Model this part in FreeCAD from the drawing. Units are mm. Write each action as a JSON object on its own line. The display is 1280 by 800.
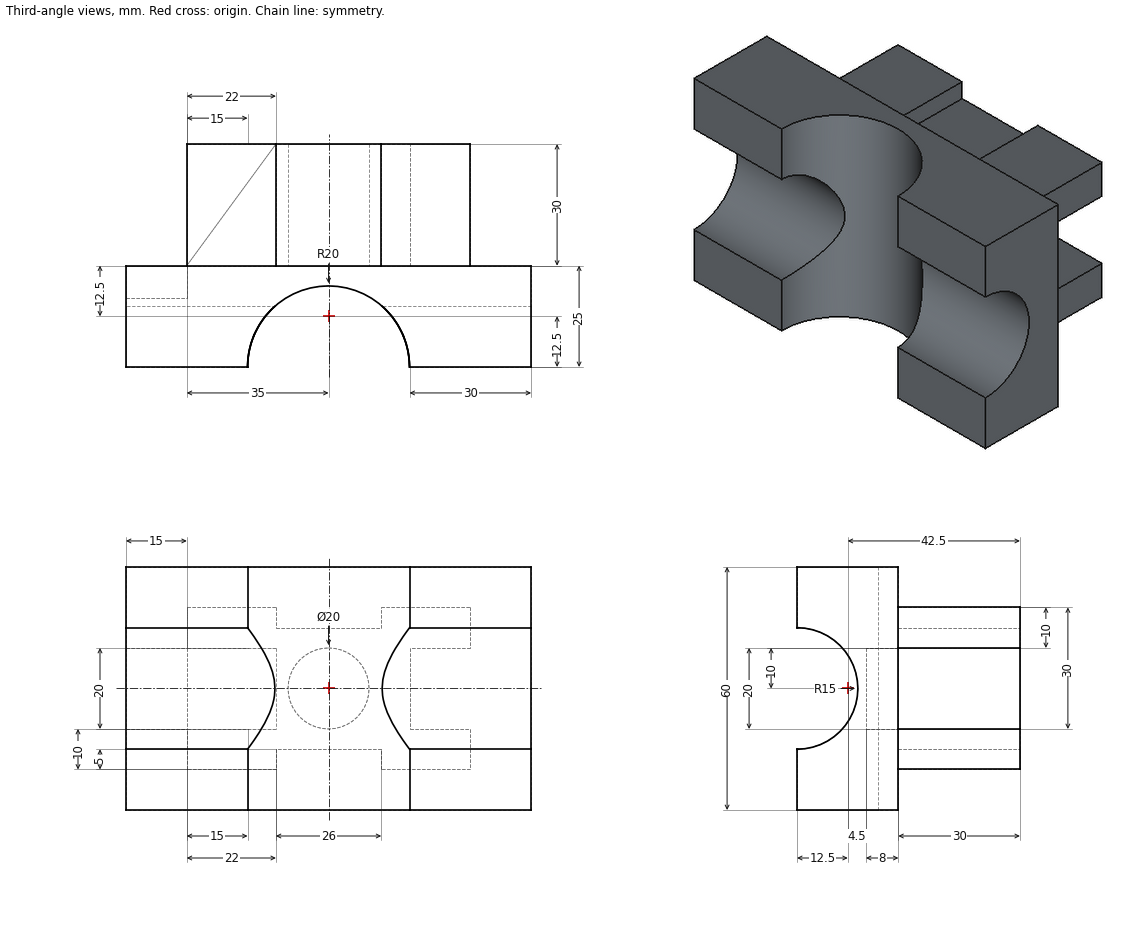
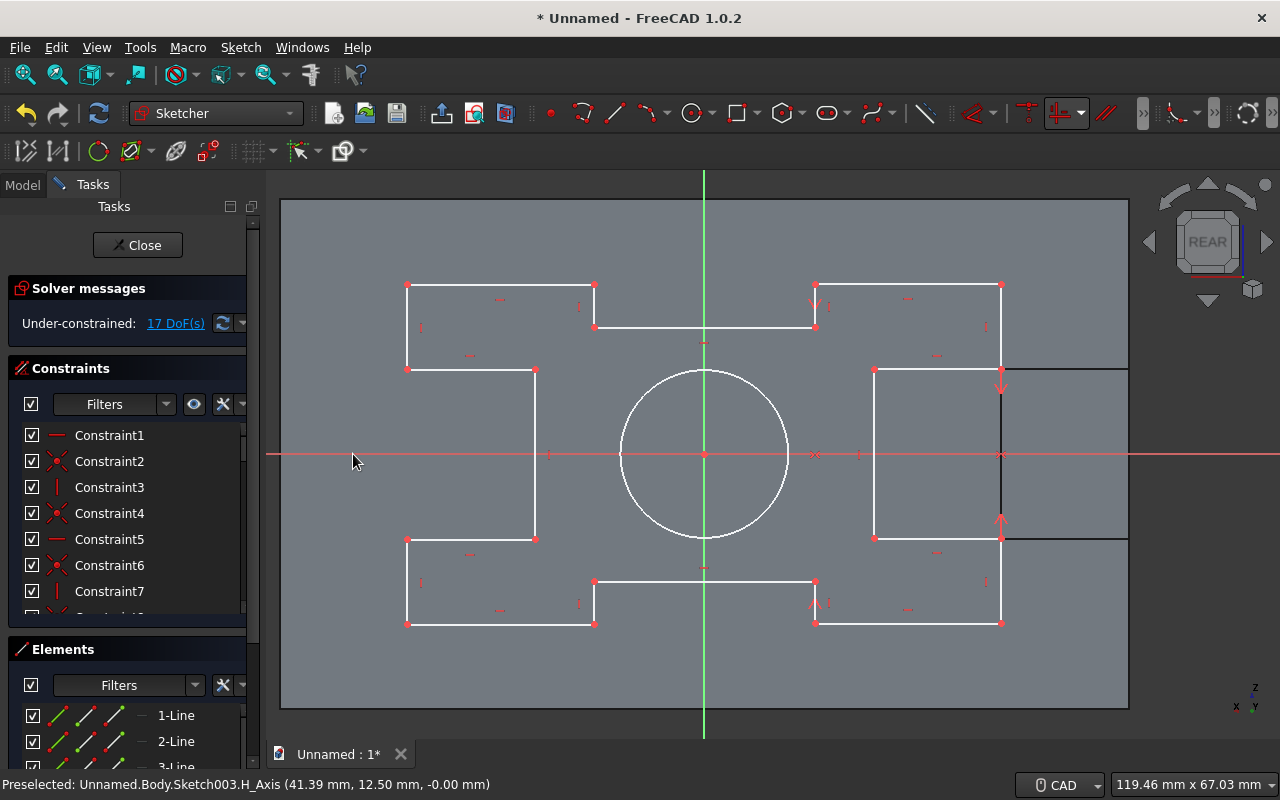
{"action": "left_click", "coordinate": [594, 582]}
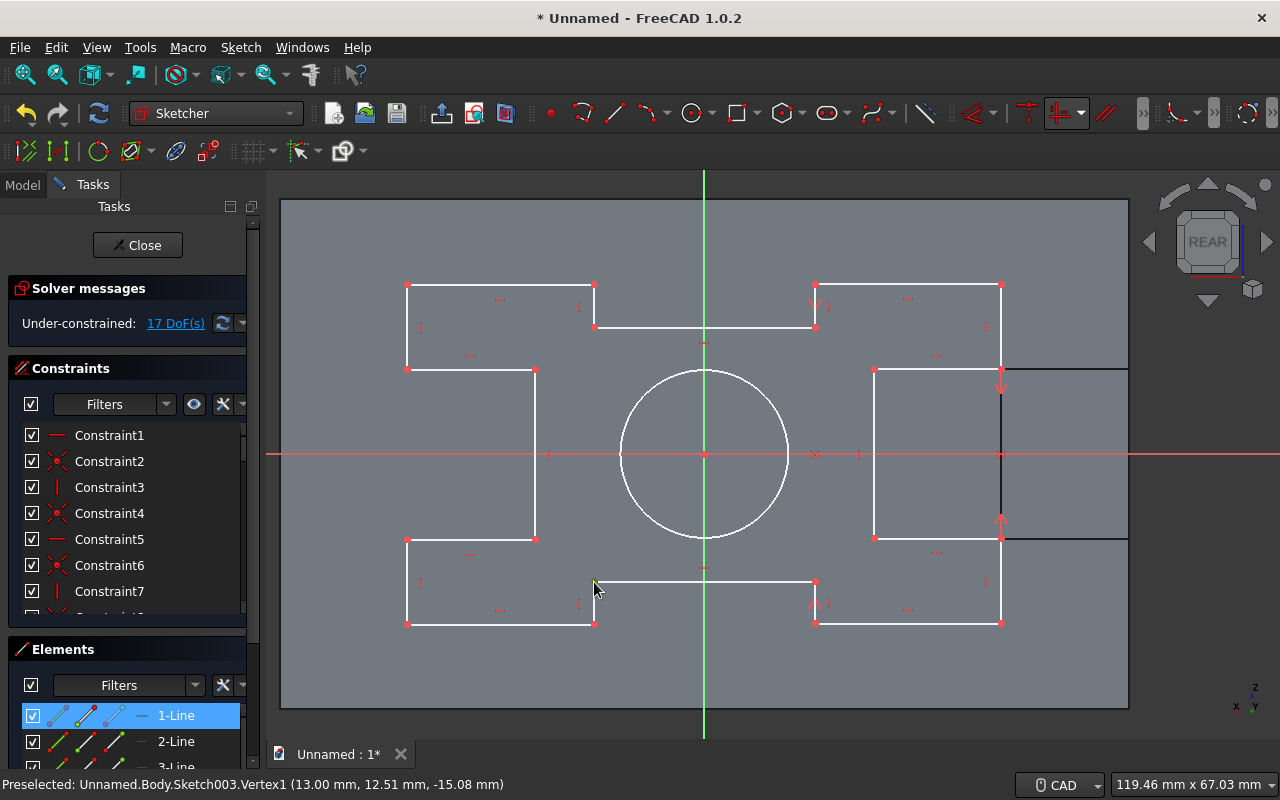
{"action": "left_click", "coordinate": [594, 328]}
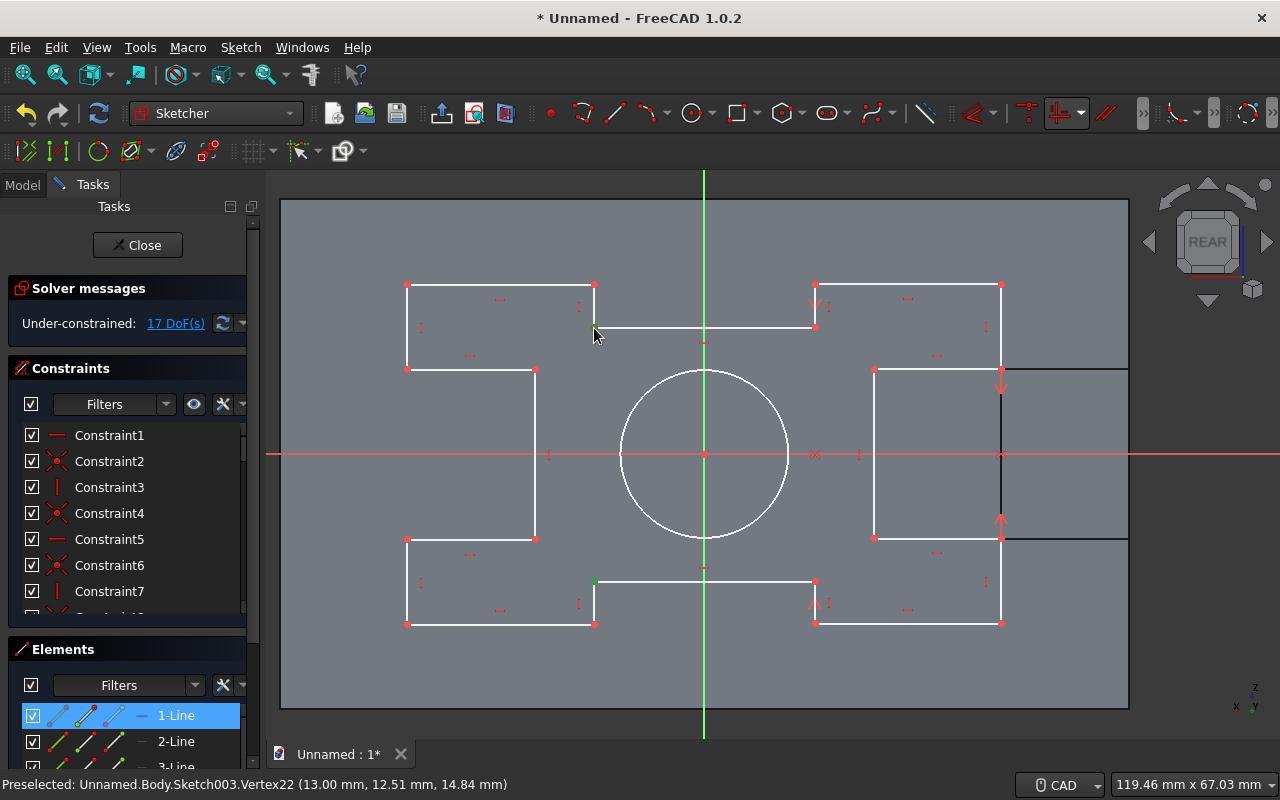
{"action": "left_click", "coordinate": [353, 454]}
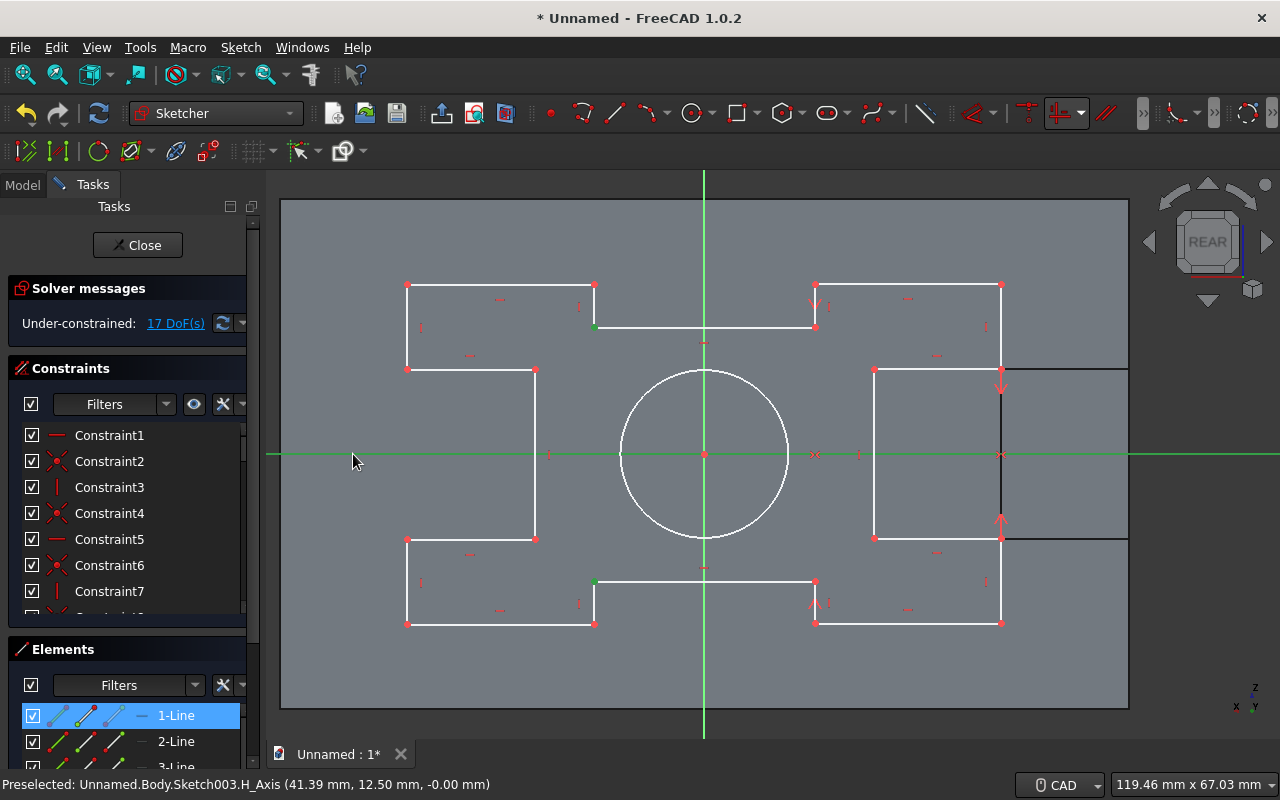
{"action": "key", "text": "s"}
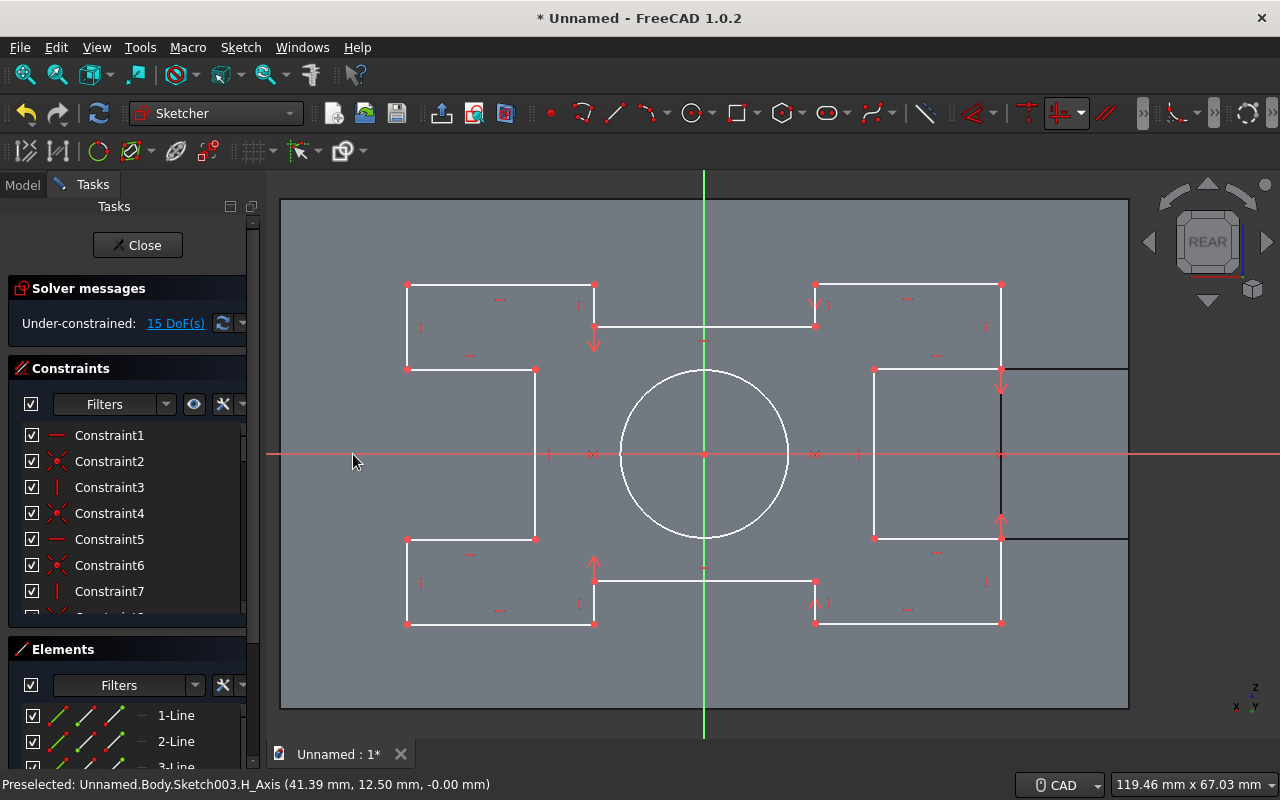
{"action": "left_click", "coordinate": [815, 284]}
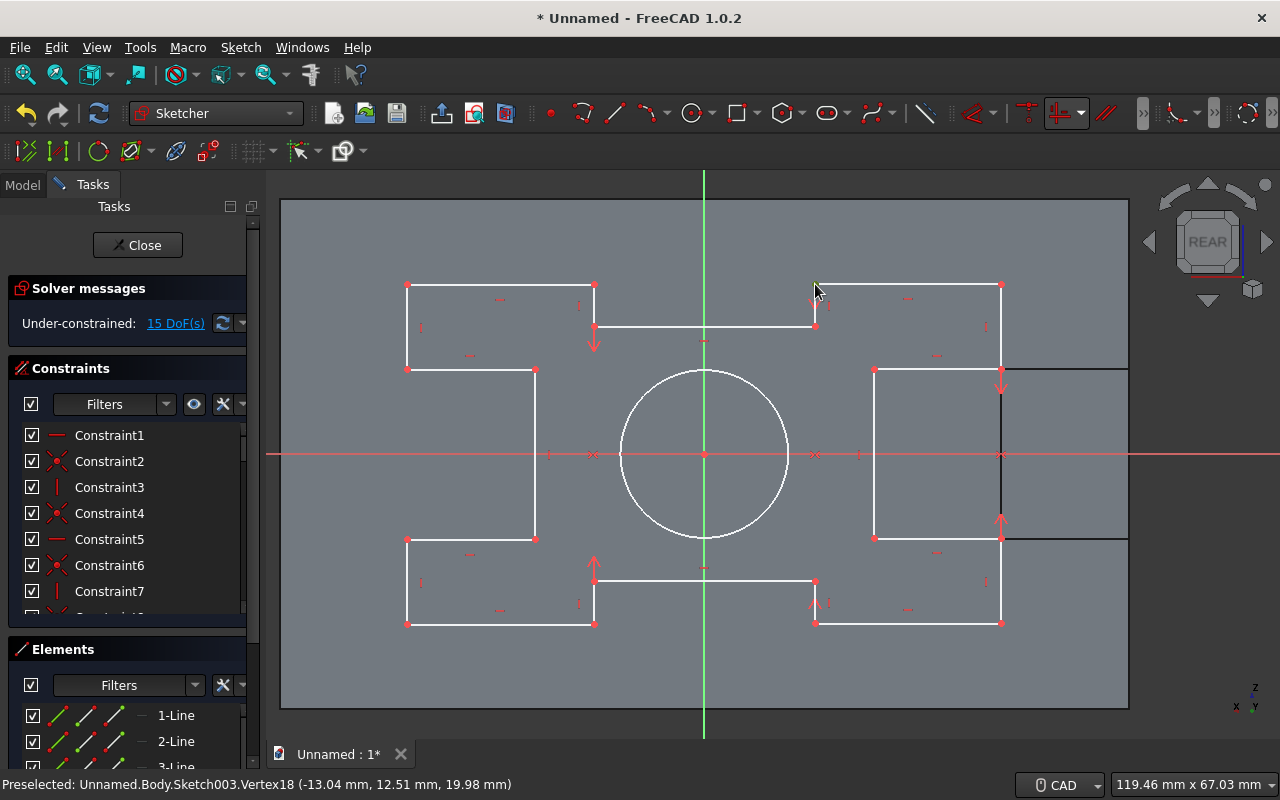
{"action": "left_click", "coordinate": [594, 285]}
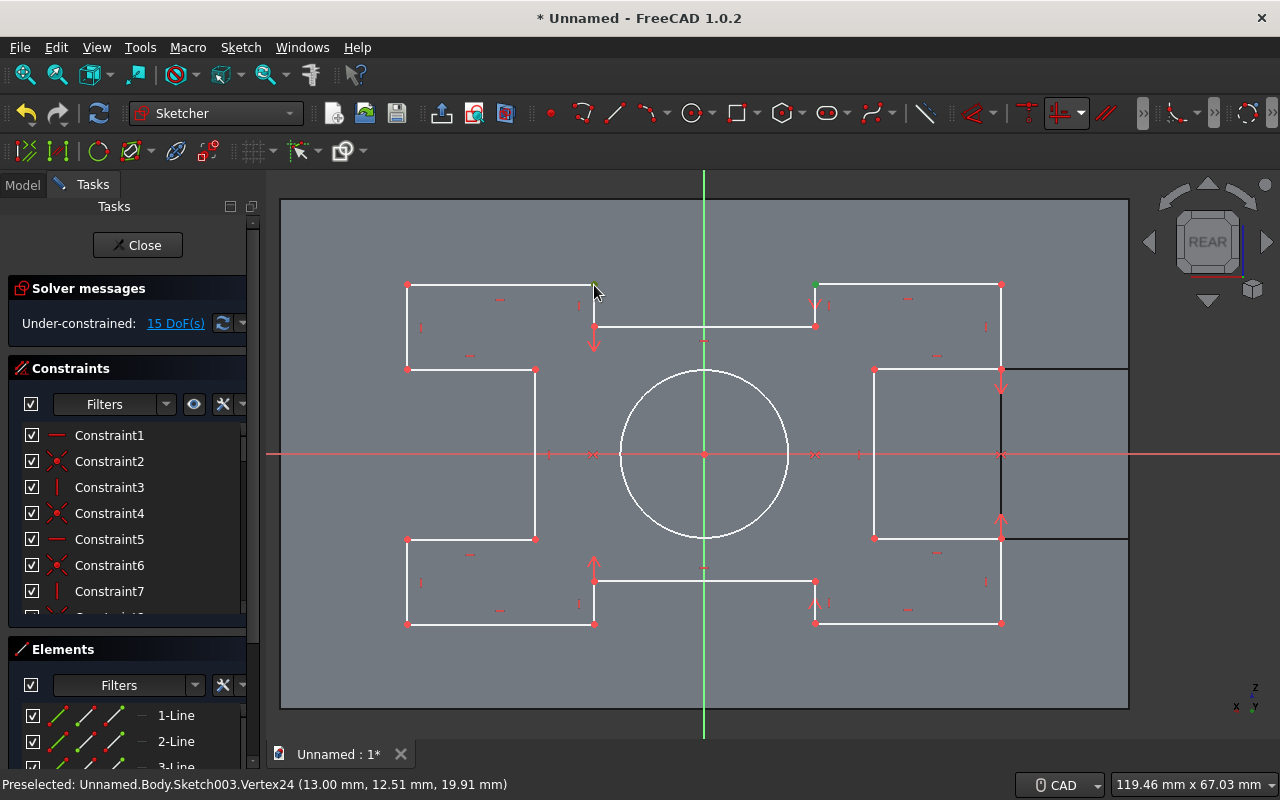
{"action": "left_click", "coordinate": [704, 674]}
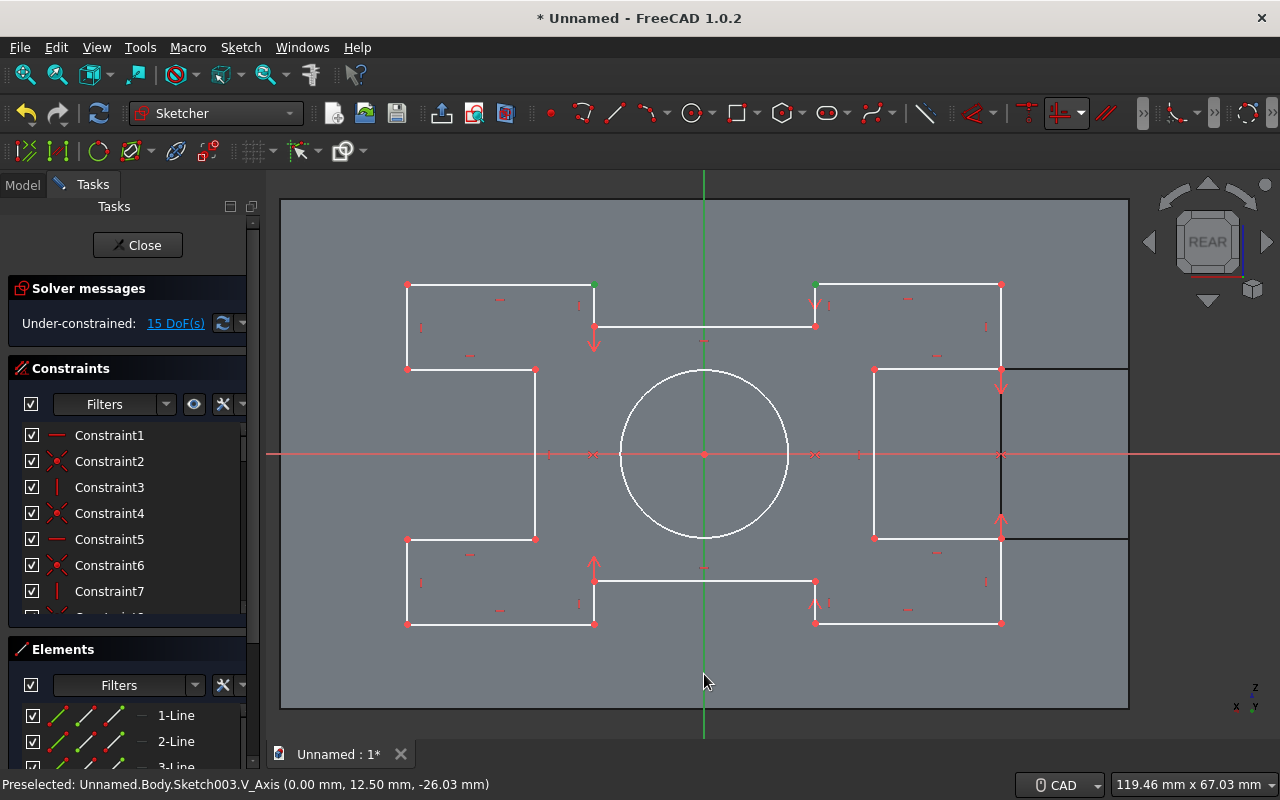
{"action": "key", "text": "s"}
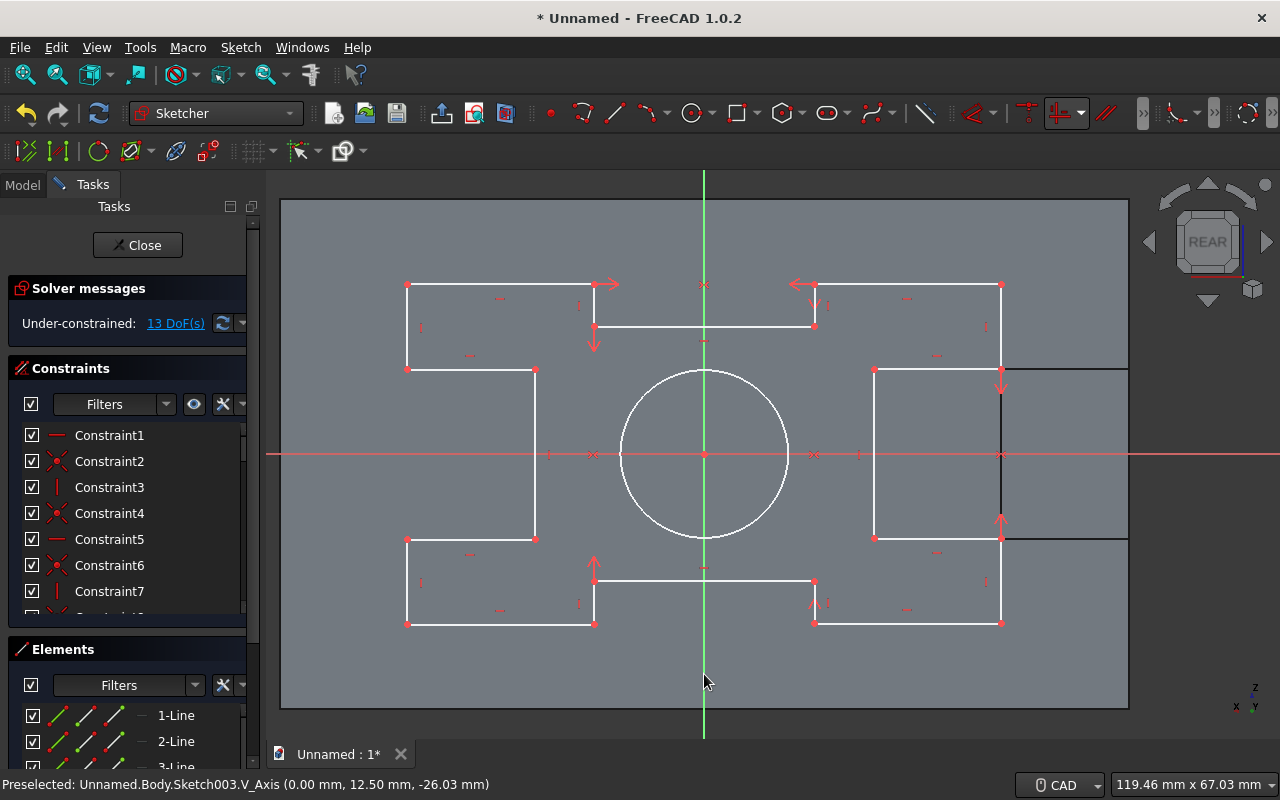
{"action": "left_click", "coordinate": [1001, 369]}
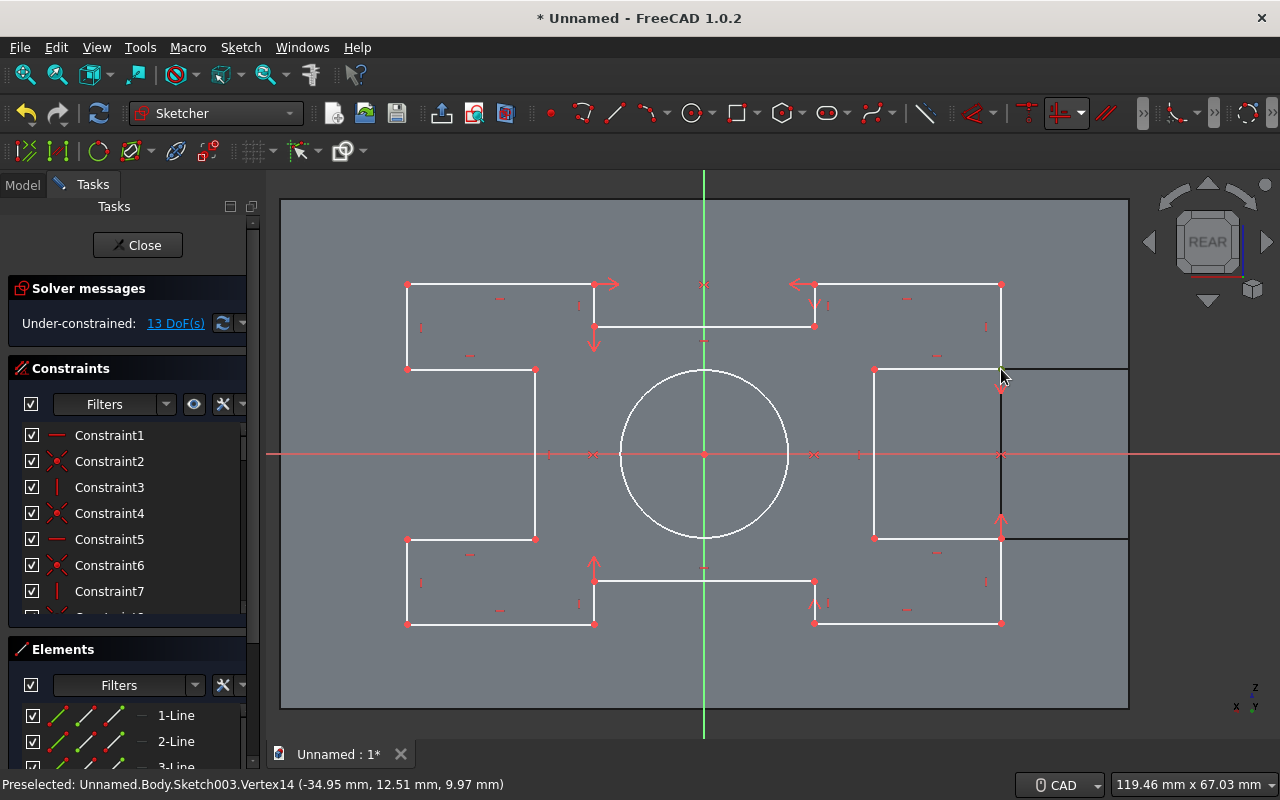
{"action": "left_click", "coordinate": [407, 370]}